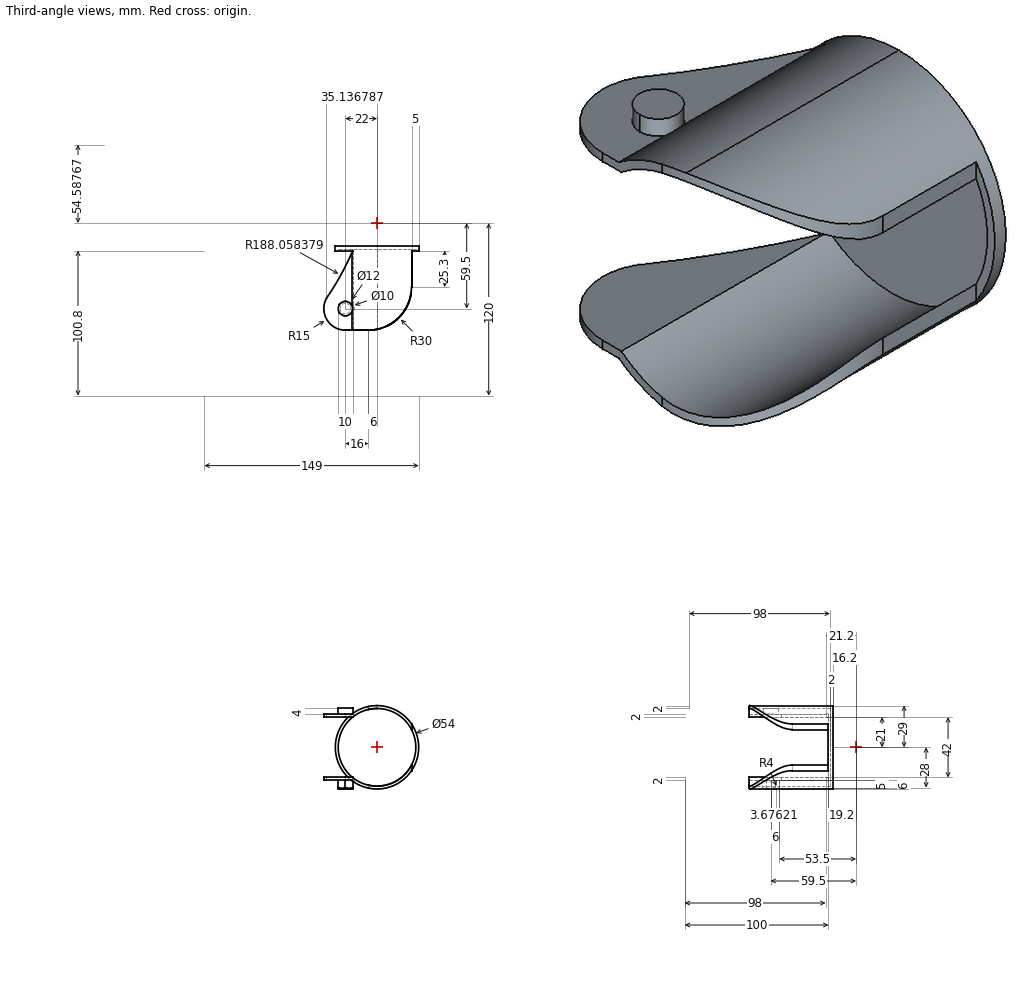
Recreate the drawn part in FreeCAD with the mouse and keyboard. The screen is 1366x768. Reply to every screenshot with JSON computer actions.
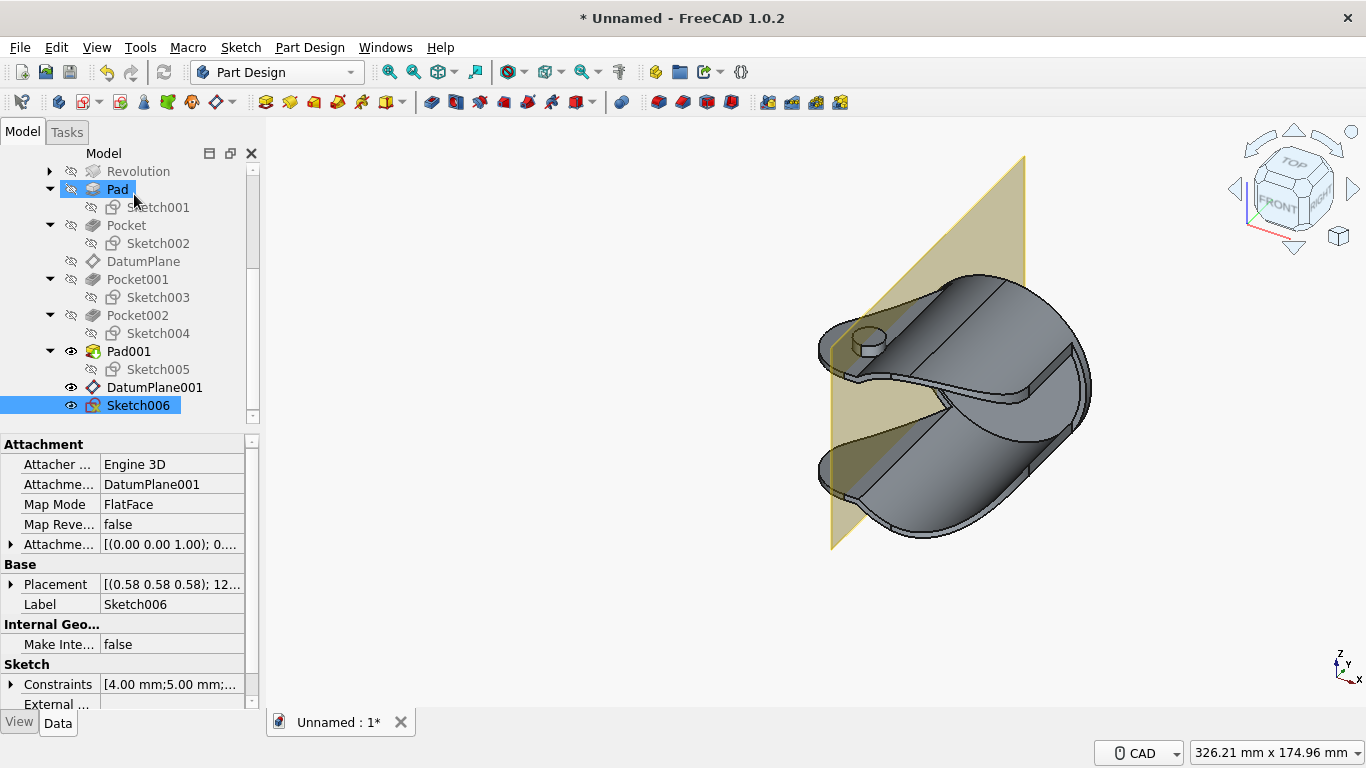
{"action": "left_click", "coordinate": [290, 102]}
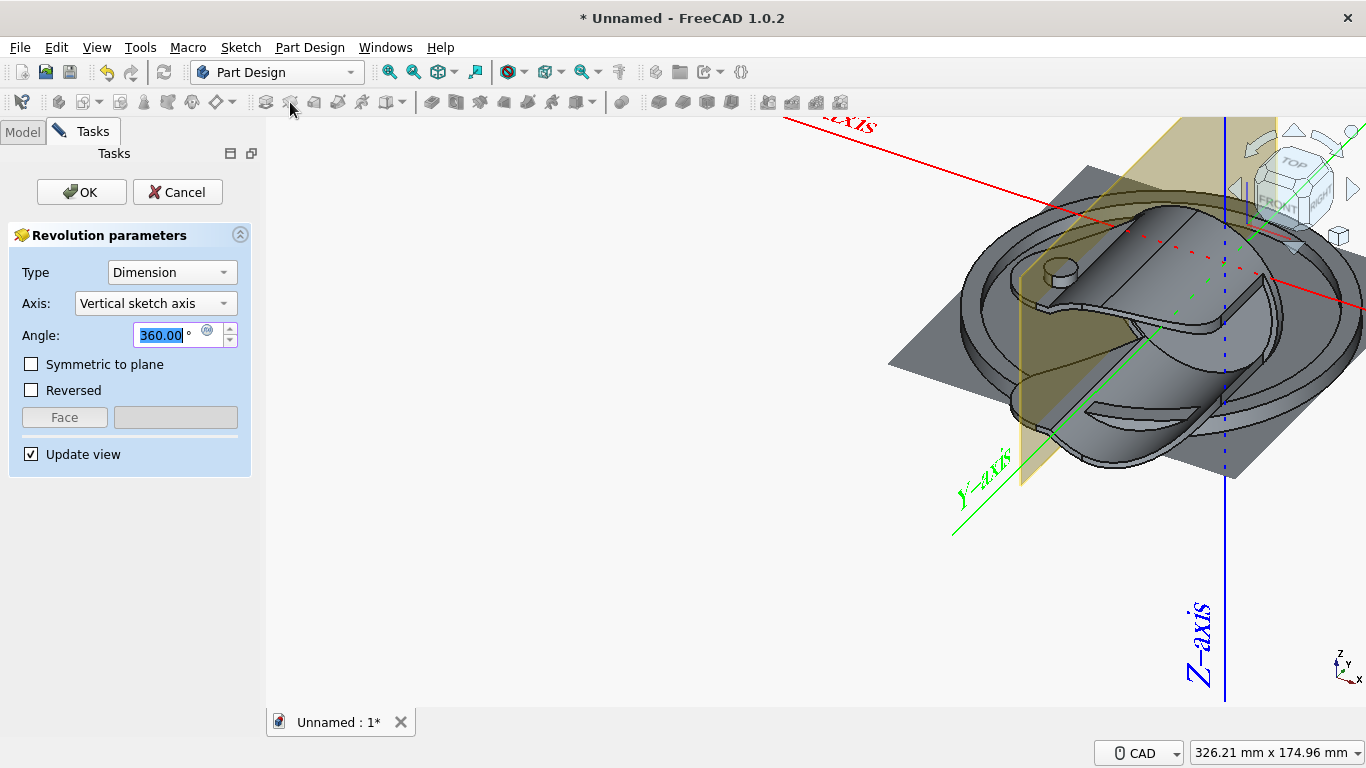
{"action": "left_click", "coordinate": [156, 304]}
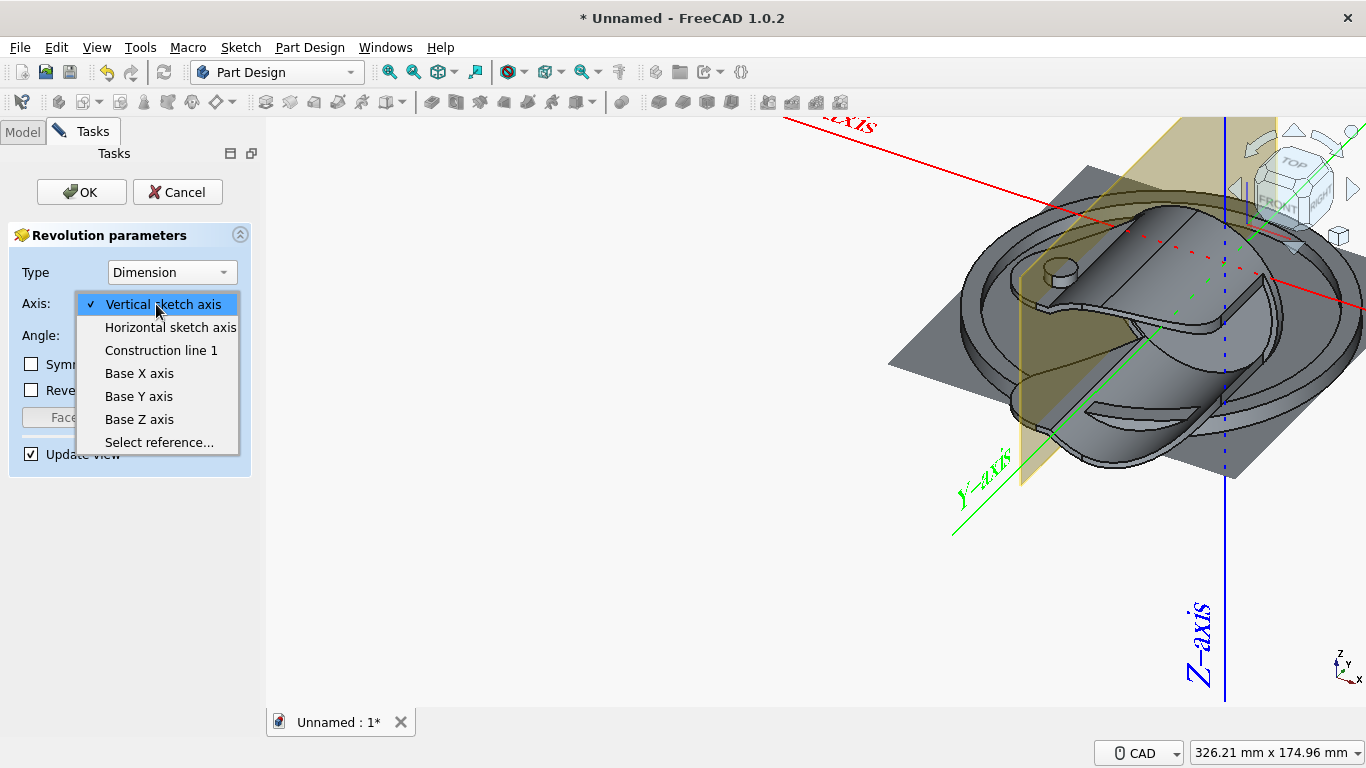
{"action": "left_click", "coordinate": [156, 350]}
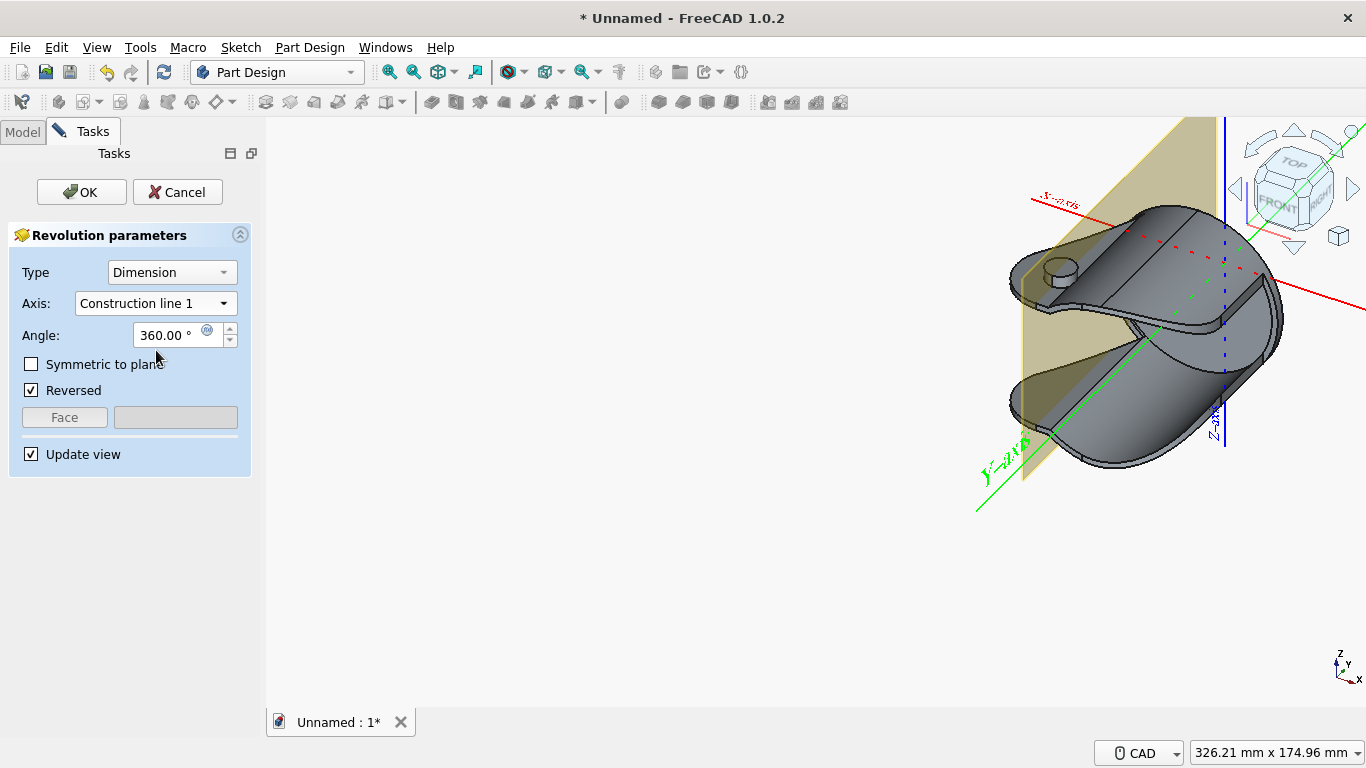
{"action": "left_click", "coordinate": [82, 192]}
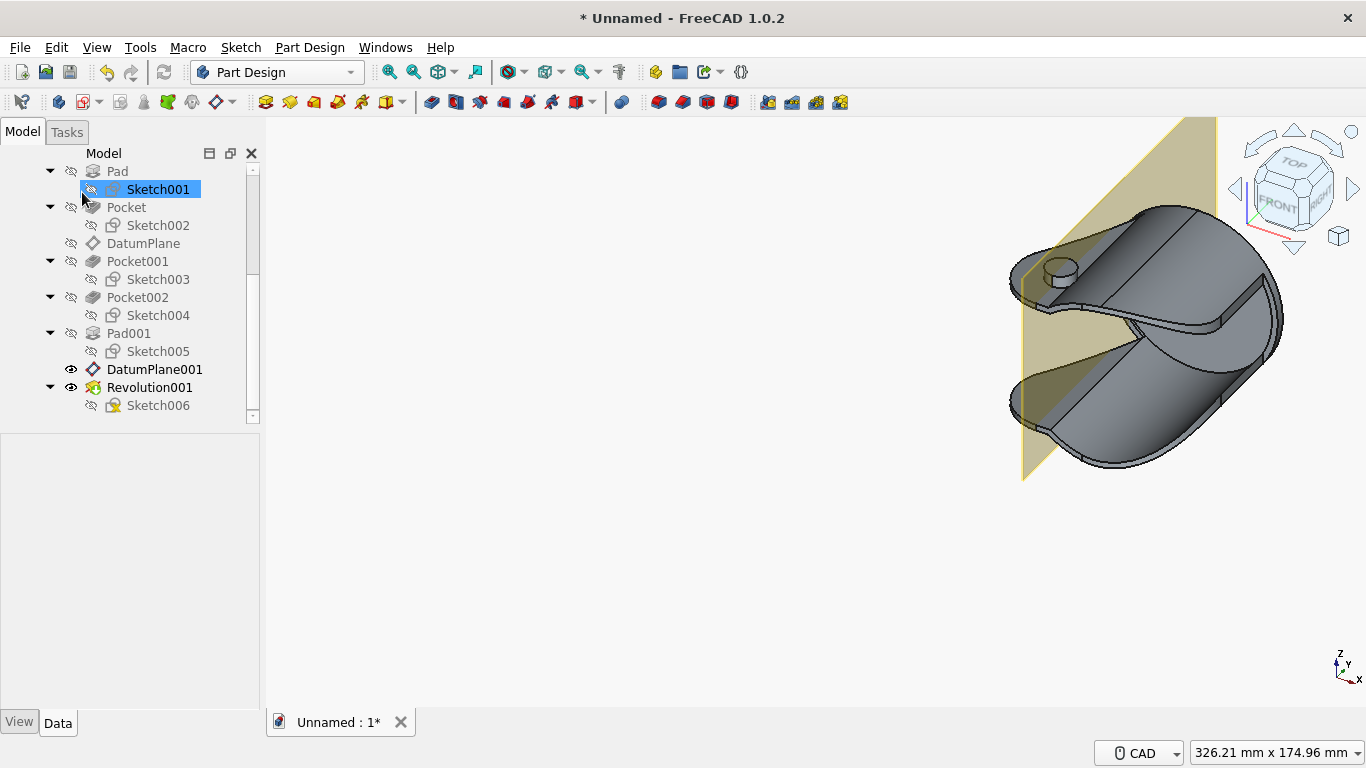
{"action": "left_click", "coordinate": [116, 369]}
{"action": "key", "text": "space"}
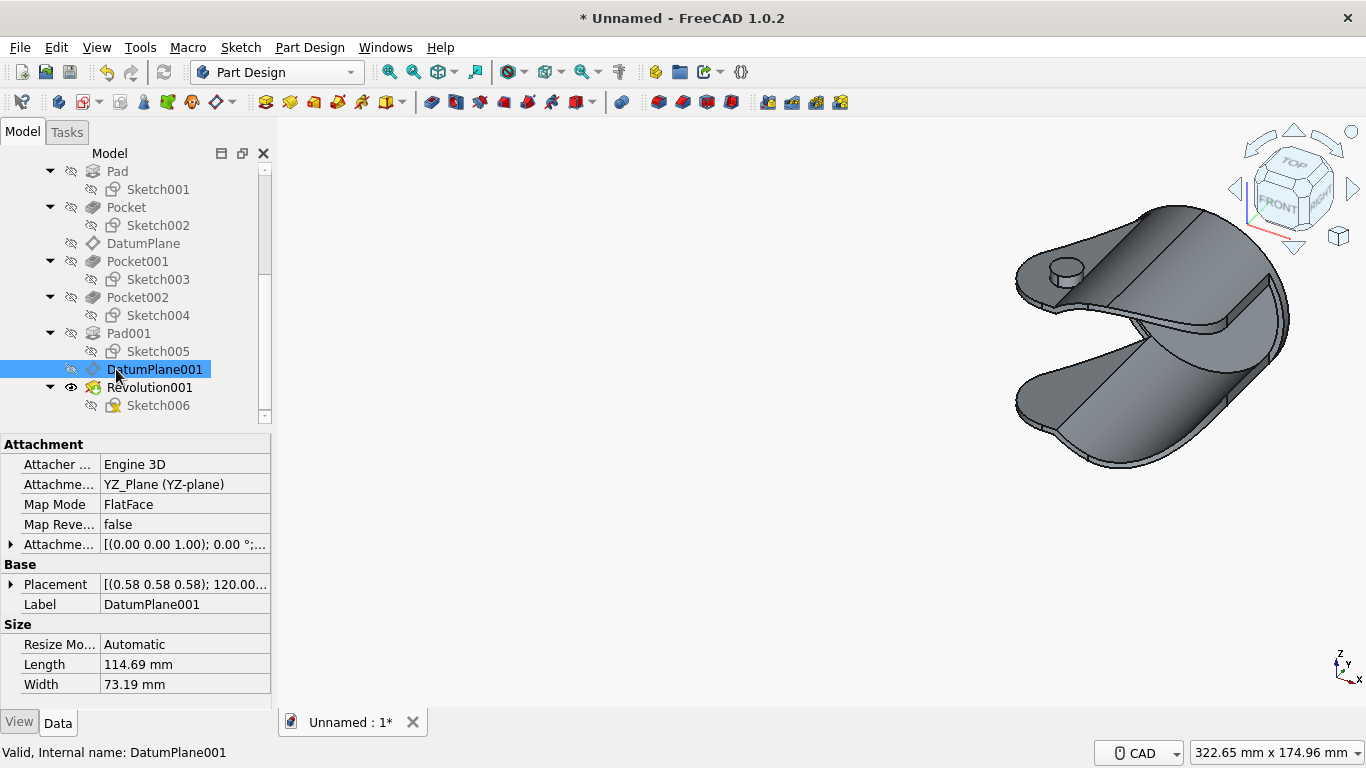
{"action": "scroll", "coordinate": [140, 293], "scroll_direction": "down", "scroll_amount": 3}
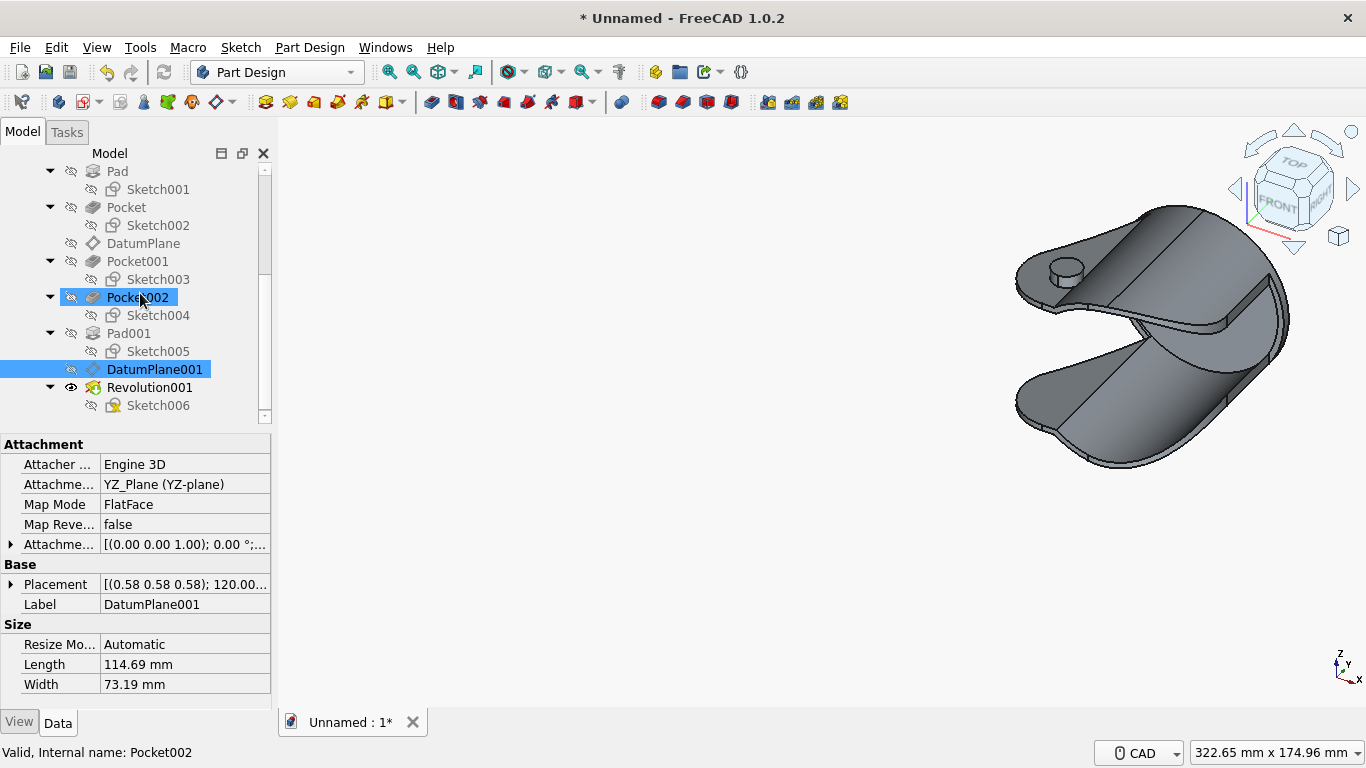
{"action": "scroll", "coordinate": [140, 293], "scroll_direction": "up", "scroll_amount": 15}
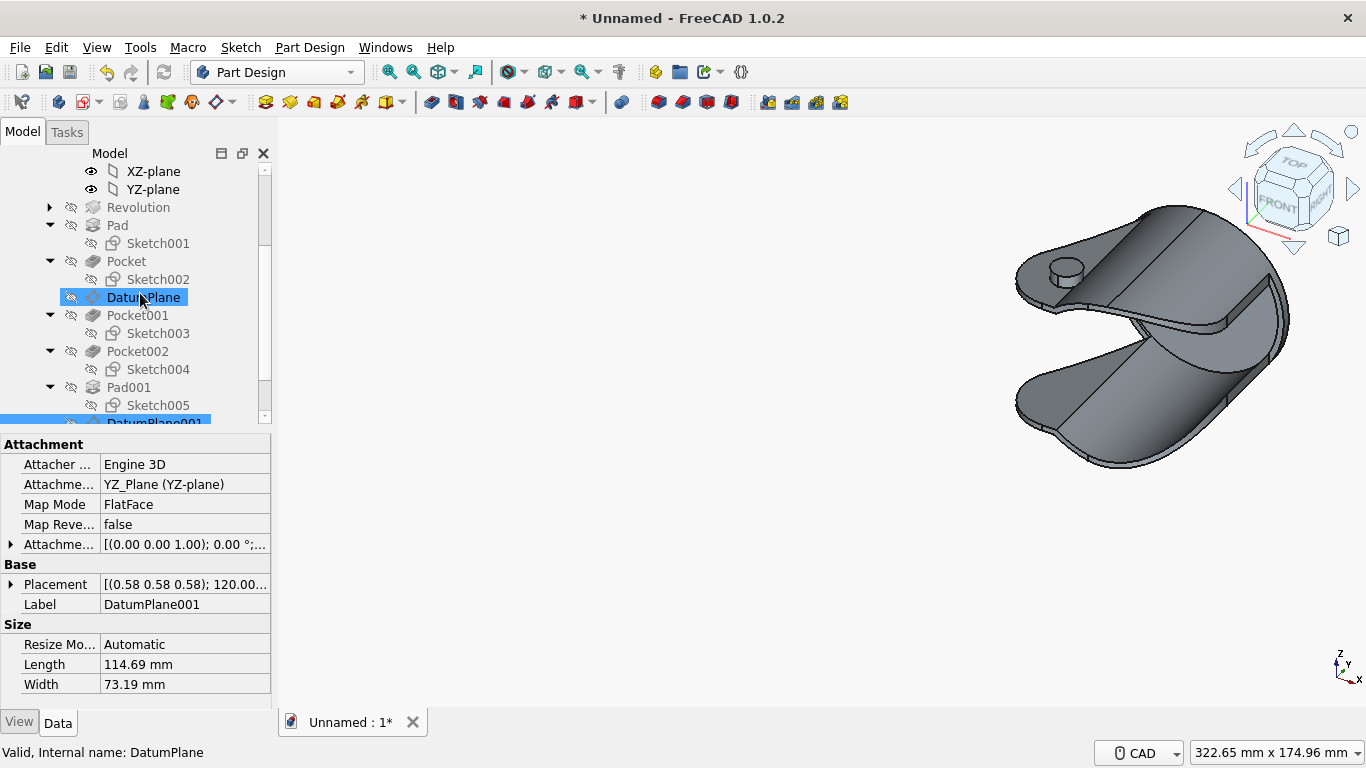
{"action": "left_click", "coordinate": [136, 279]}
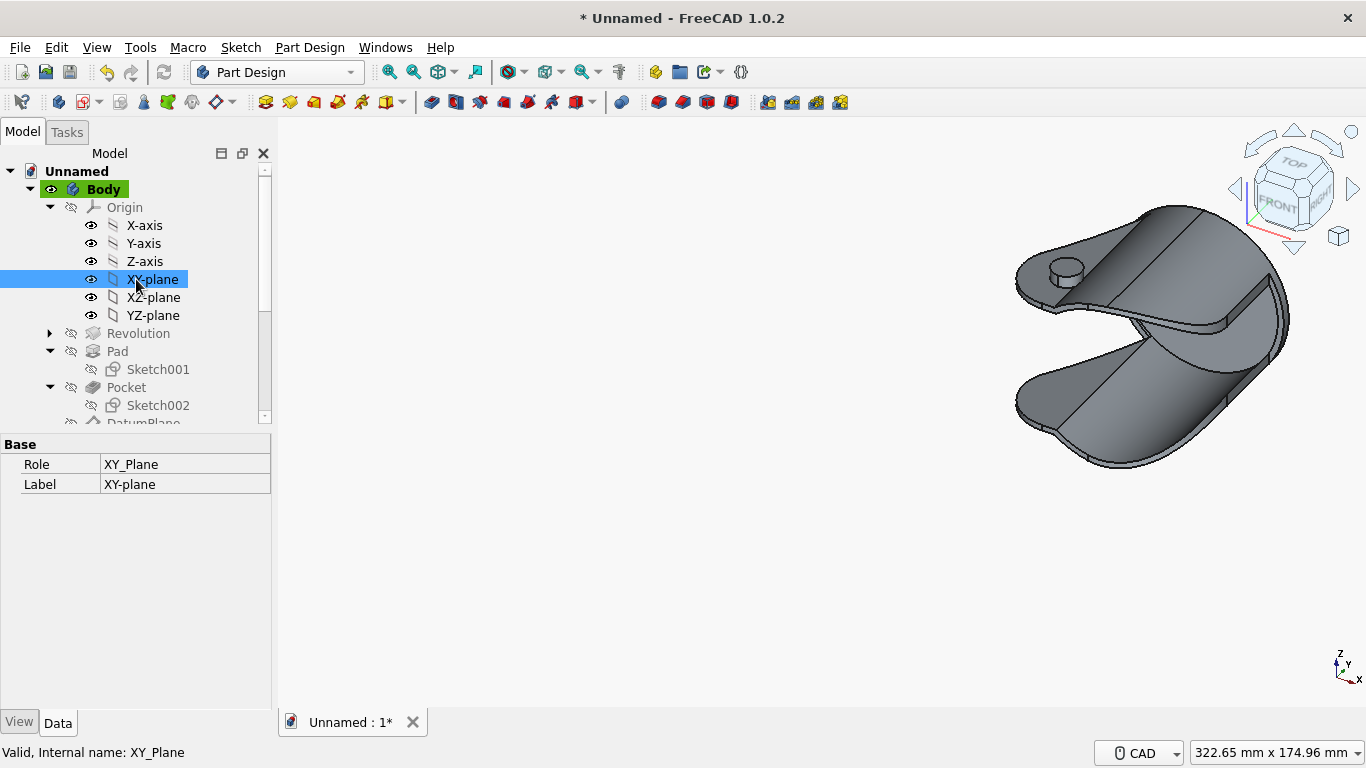
{"action": "left_click", "coordinate": [216, 102]}